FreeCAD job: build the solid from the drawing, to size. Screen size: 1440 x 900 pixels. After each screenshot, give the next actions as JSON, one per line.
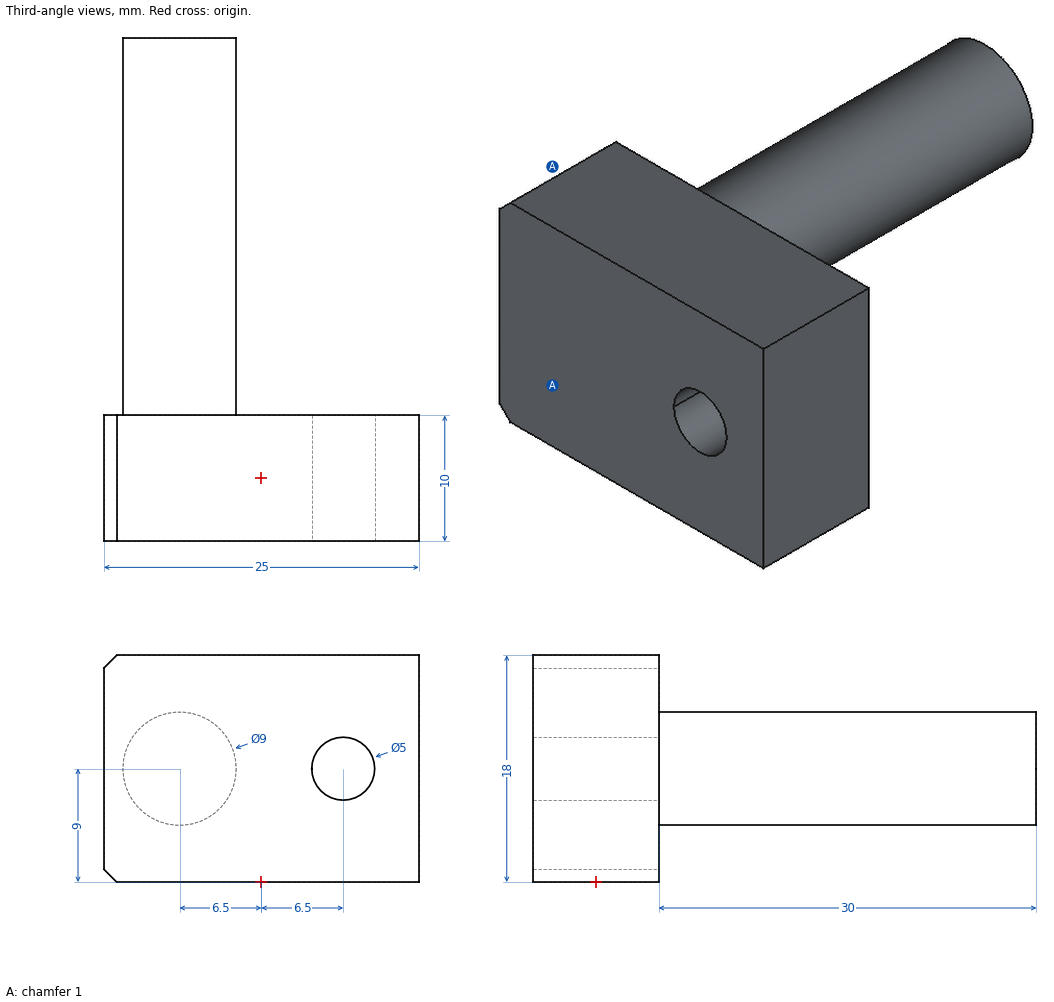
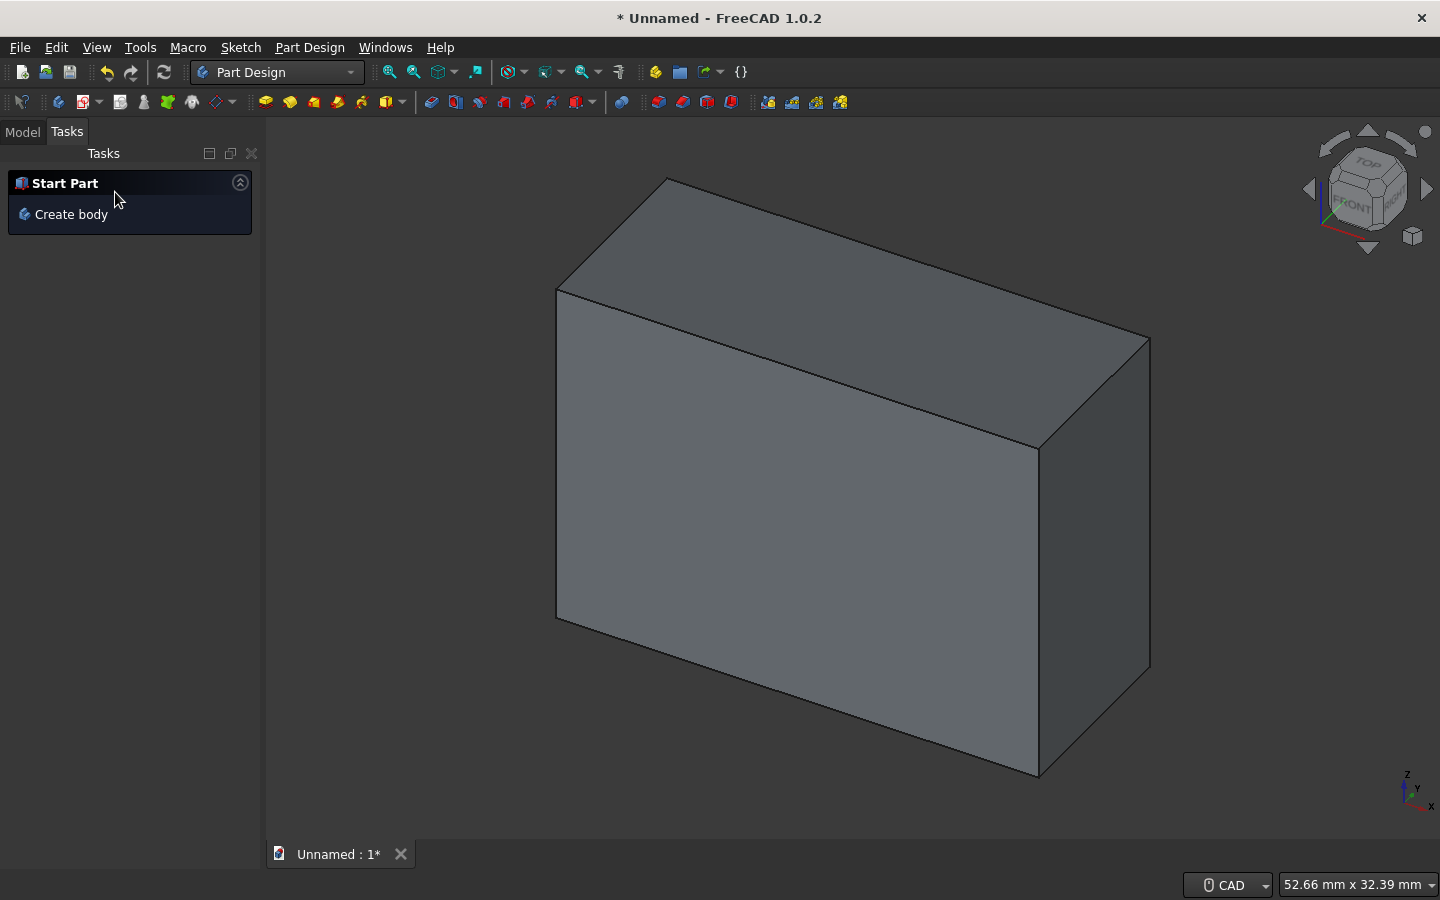
{"action": "key", "text": "4"}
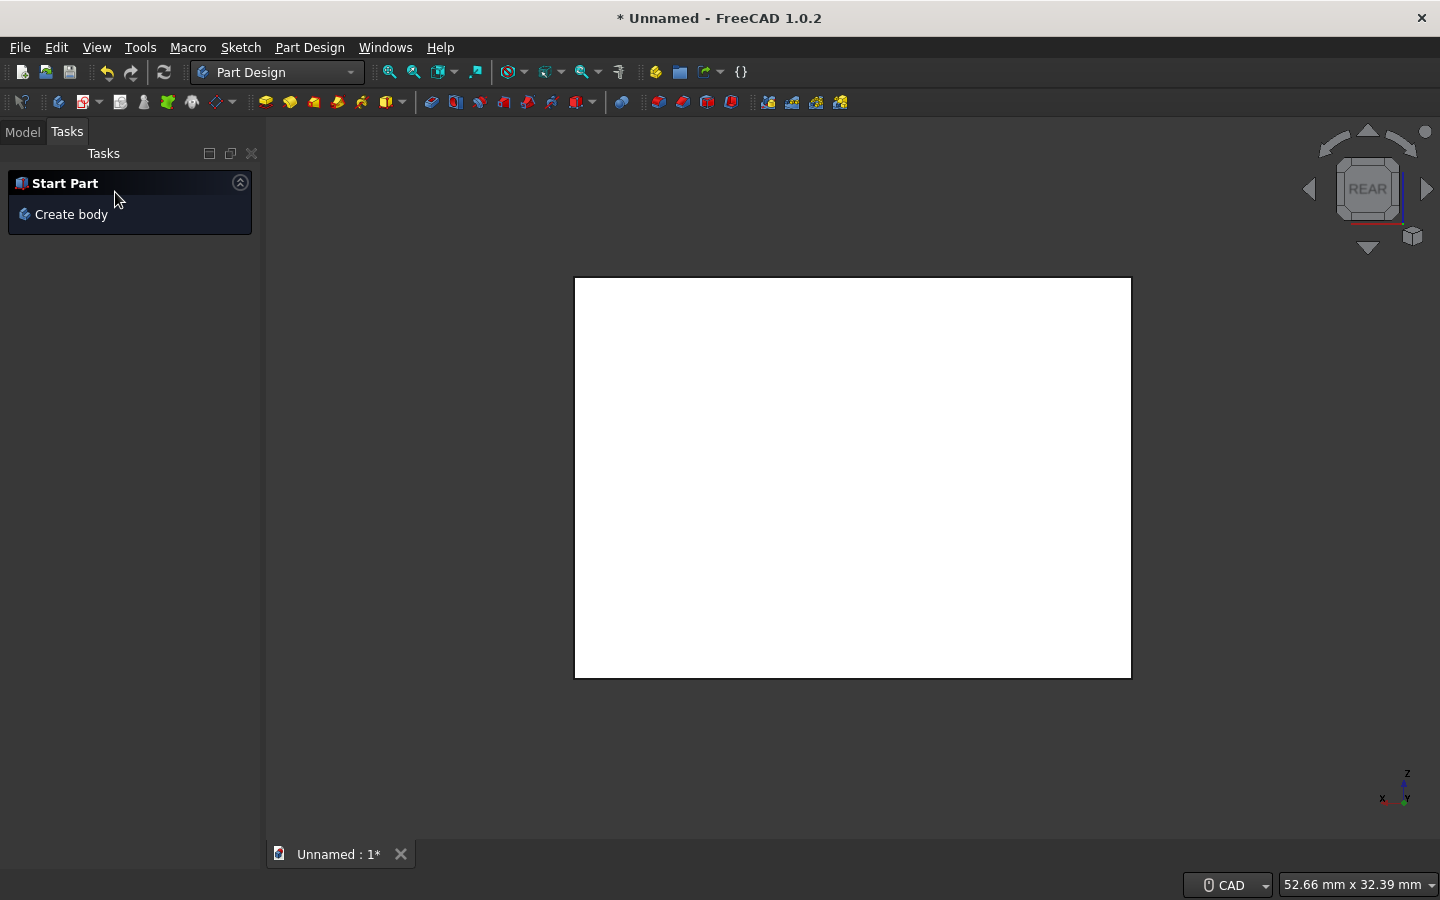
{"action": "left_click", "coordinate": [853, 477]}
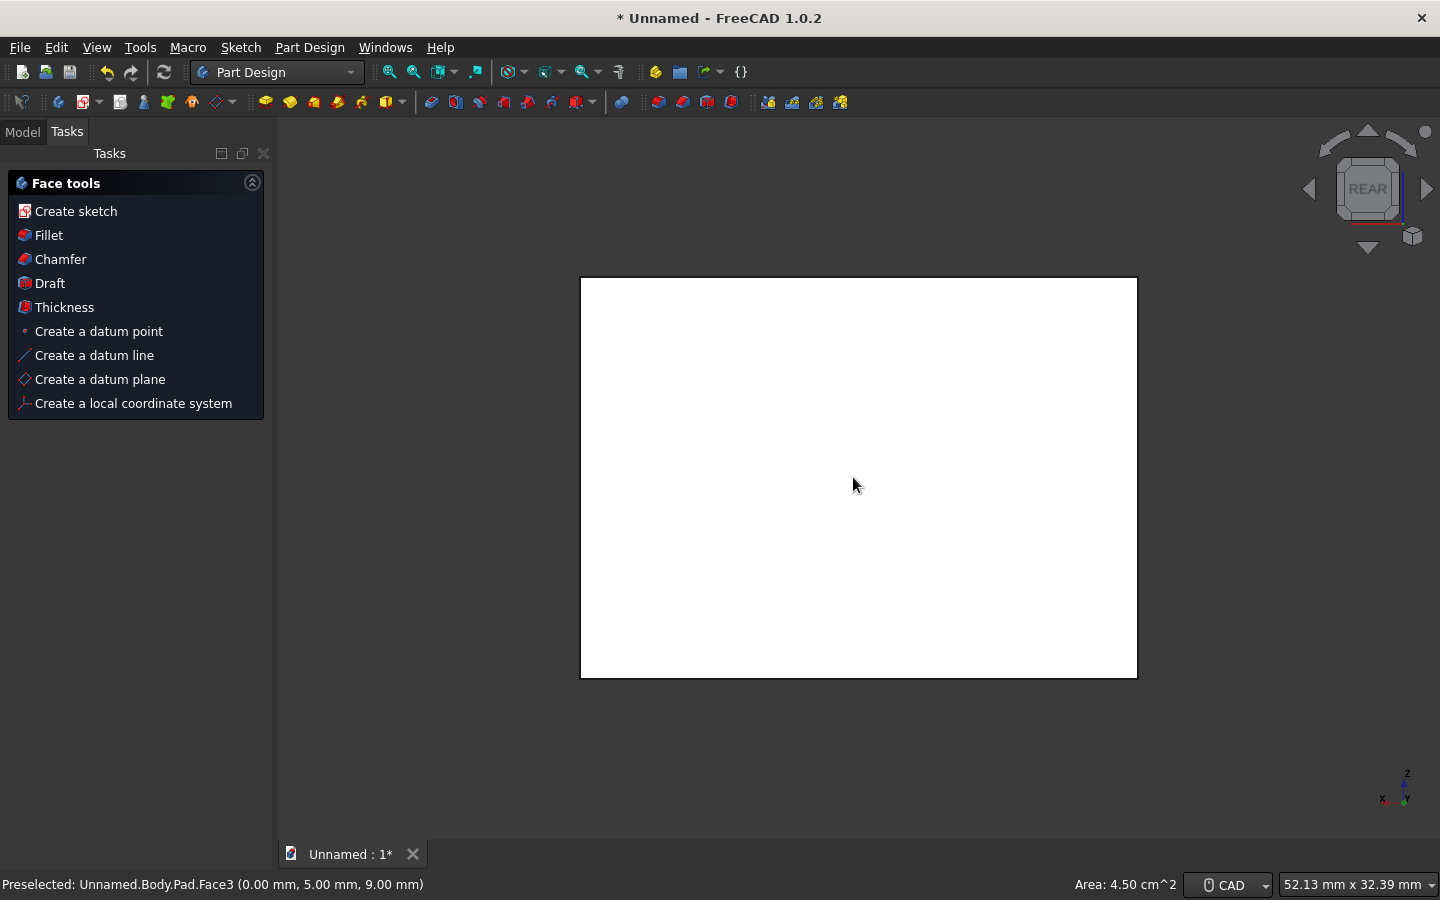
{"action": "left_click", "coordinate": [84, 102]}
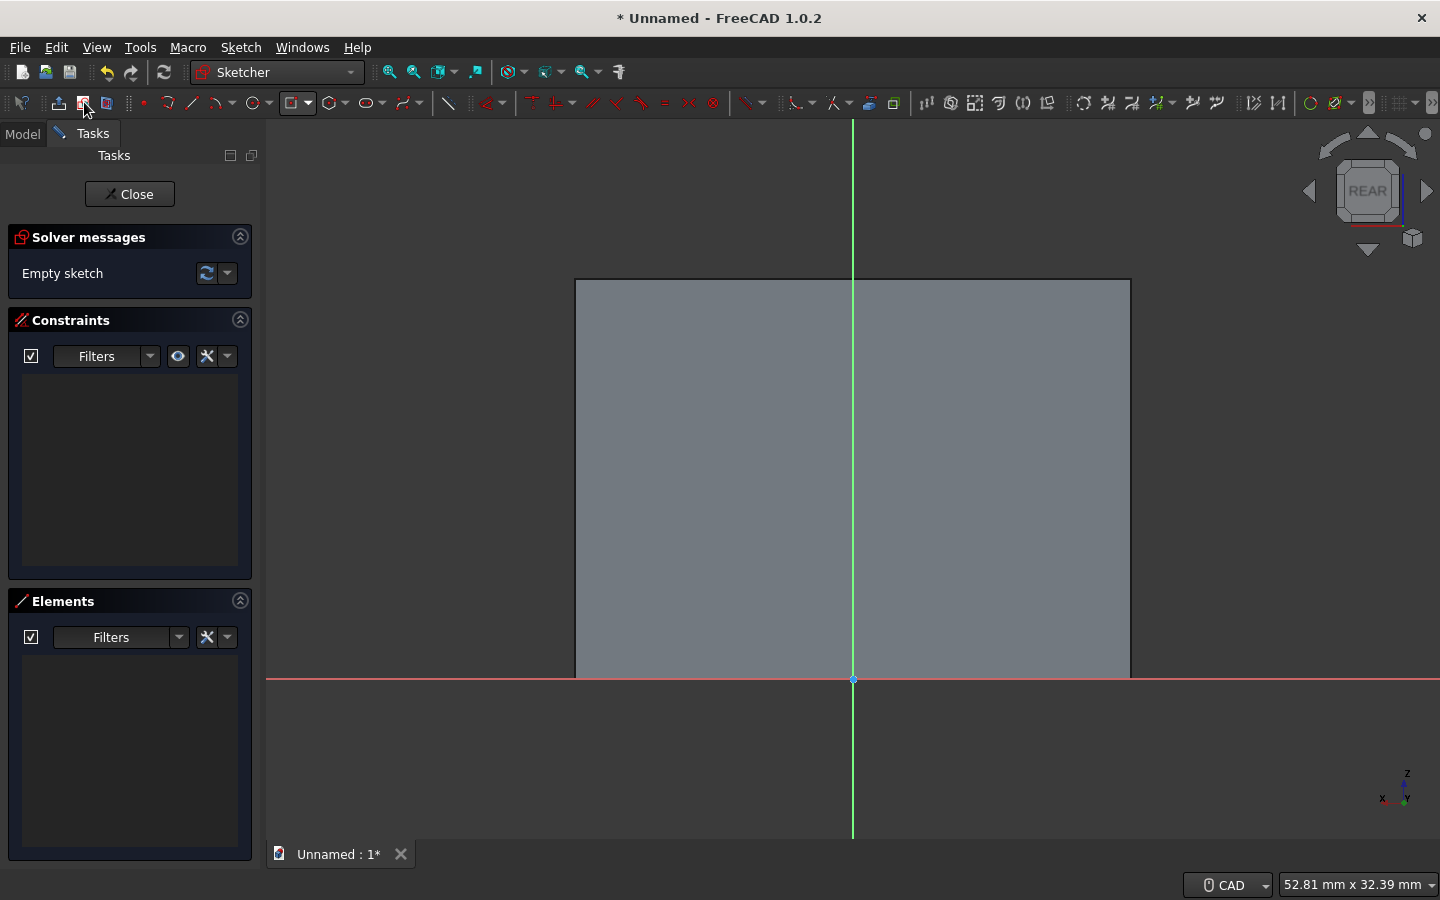
{"action": "scroll", "coordinate": [1275, 631], "scroll_direction": "up", "scroll_amount": 2}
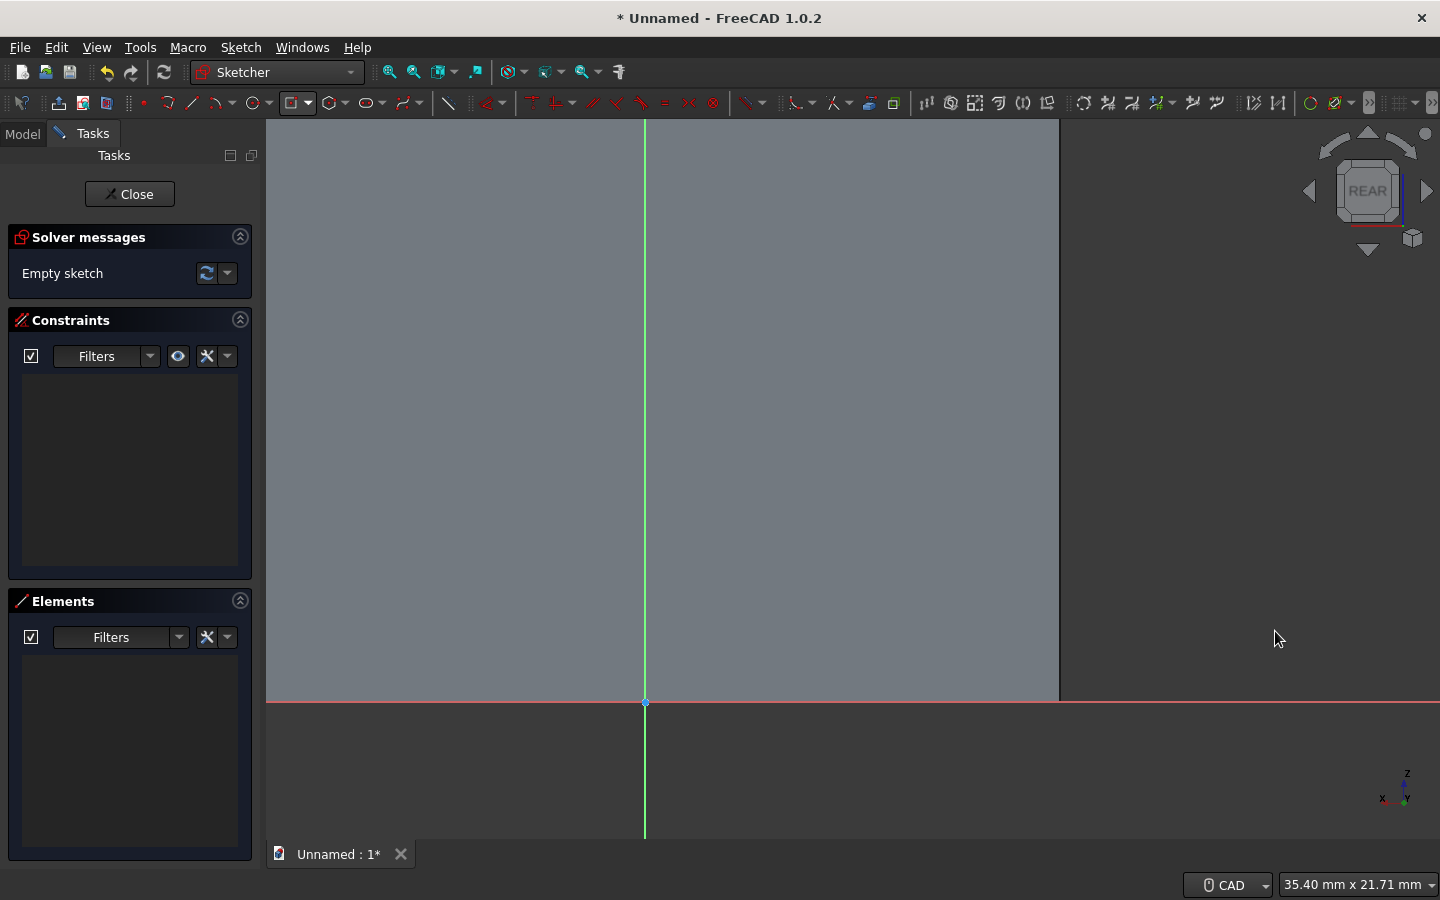
{"action": "key", "text": "g c"}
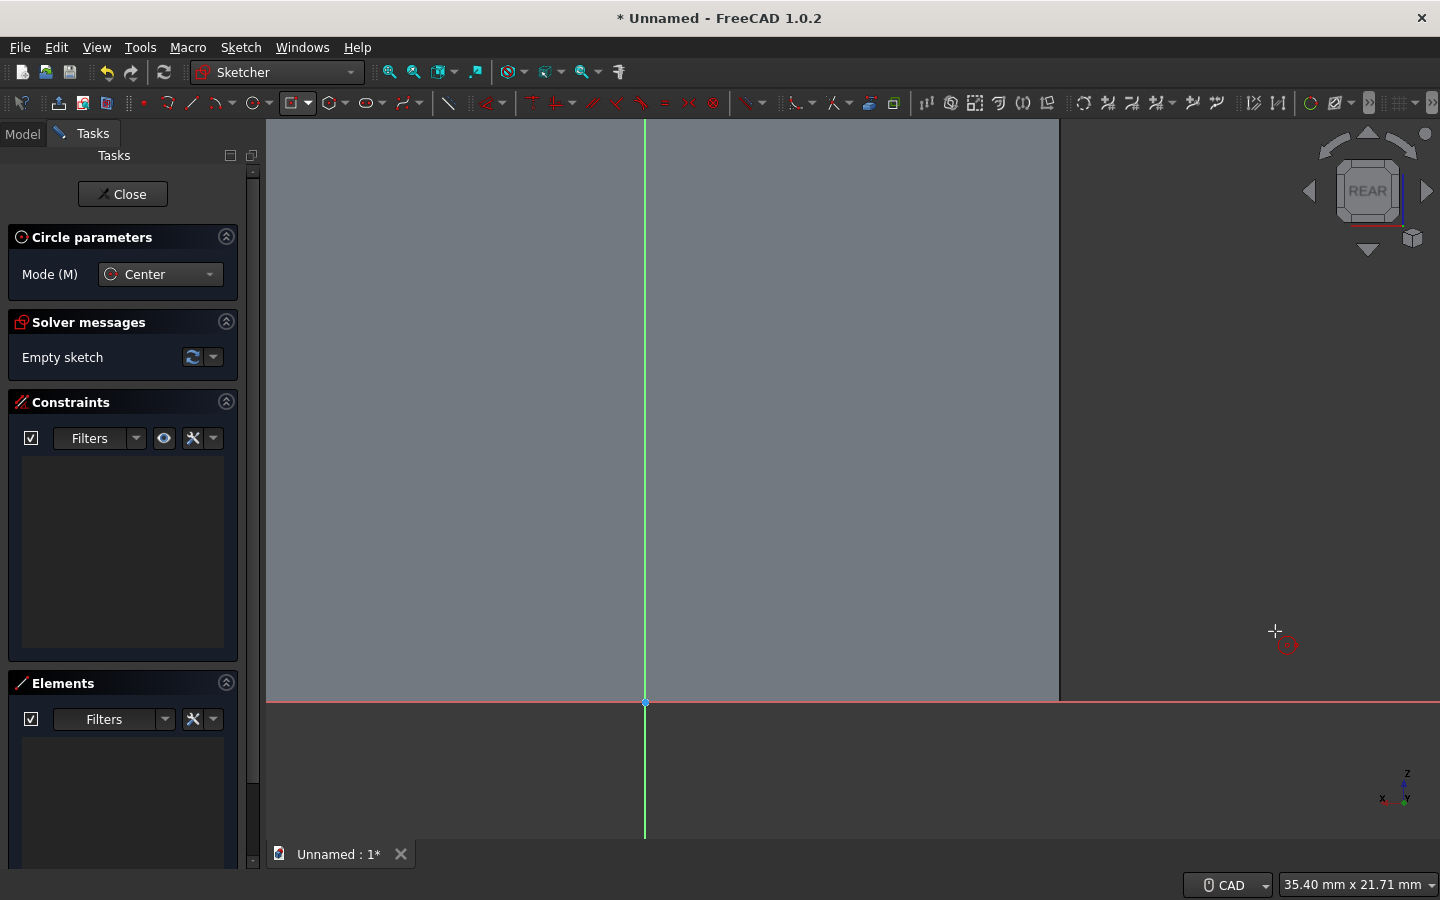
{"action": "left_click", "coordinate": [861, 404]}
{"action": "mouse_move", "coordinate": [966, 298]}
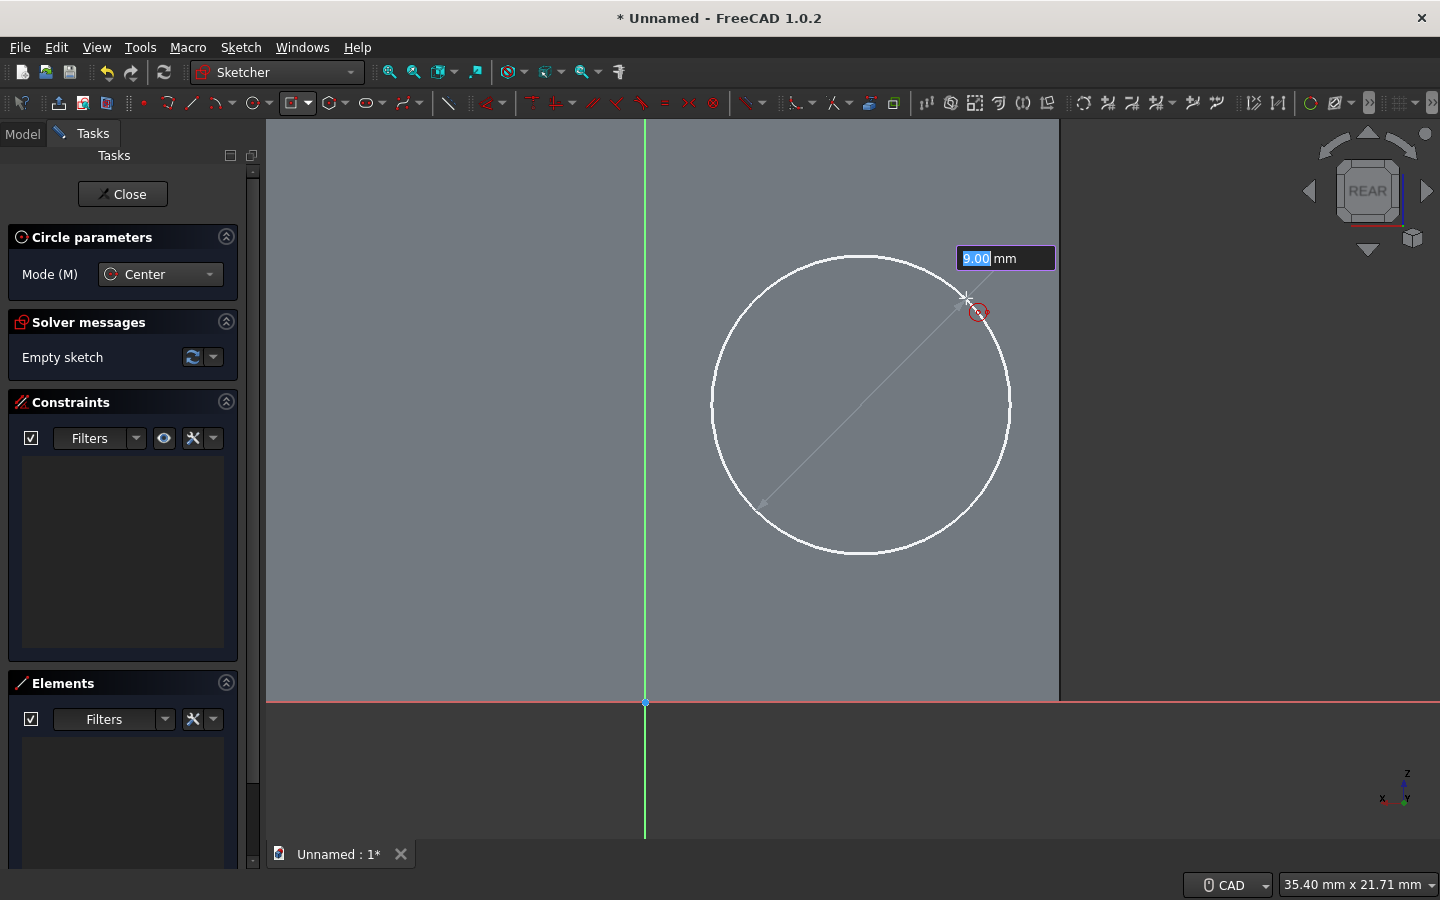
{"action": "type", "text": "9"}
{"action": "key", "text": "Return"}
{"action": "key", "text": "Escape"}